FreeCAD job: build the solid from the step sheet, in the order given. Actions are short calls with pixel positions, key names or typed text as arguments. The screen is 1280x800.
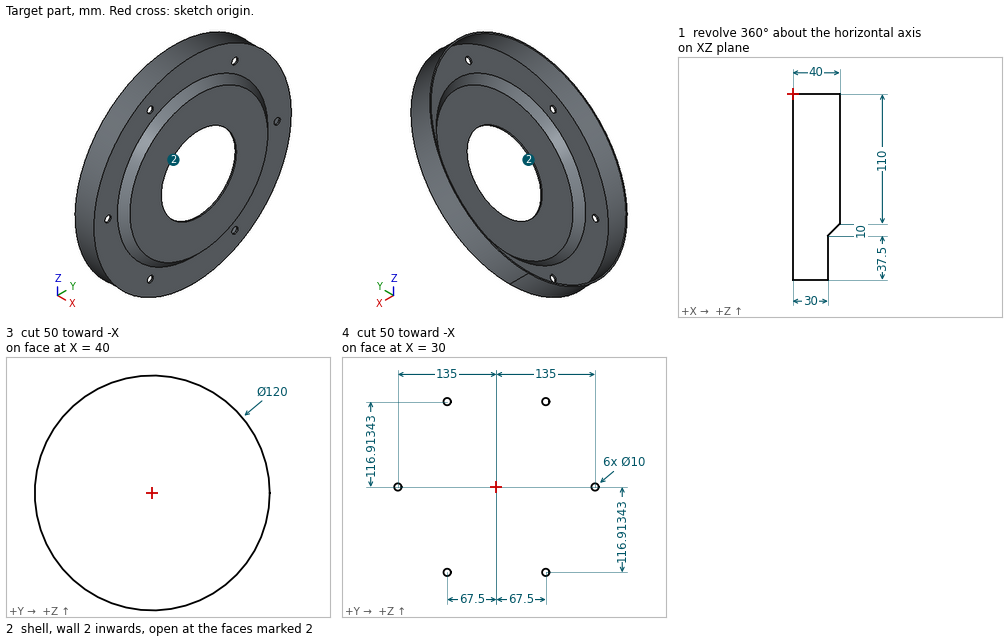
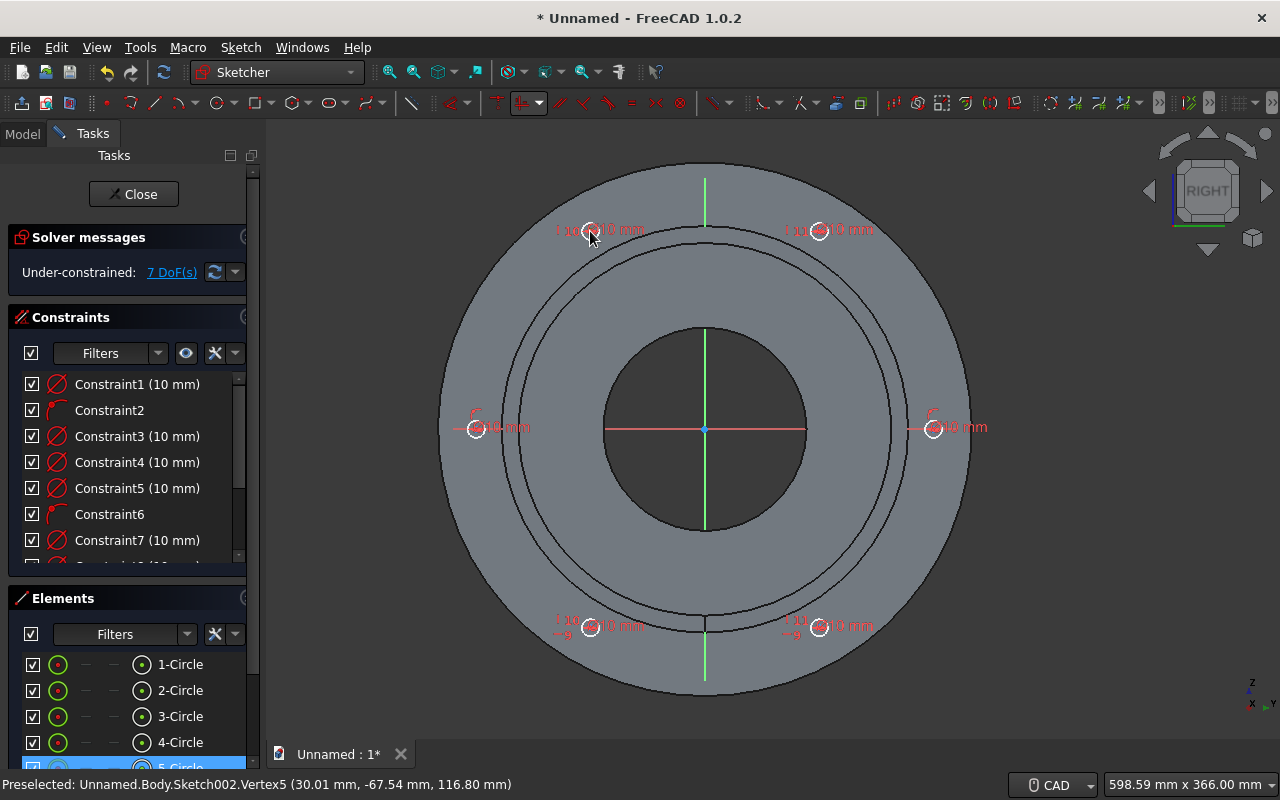
click(819, 231)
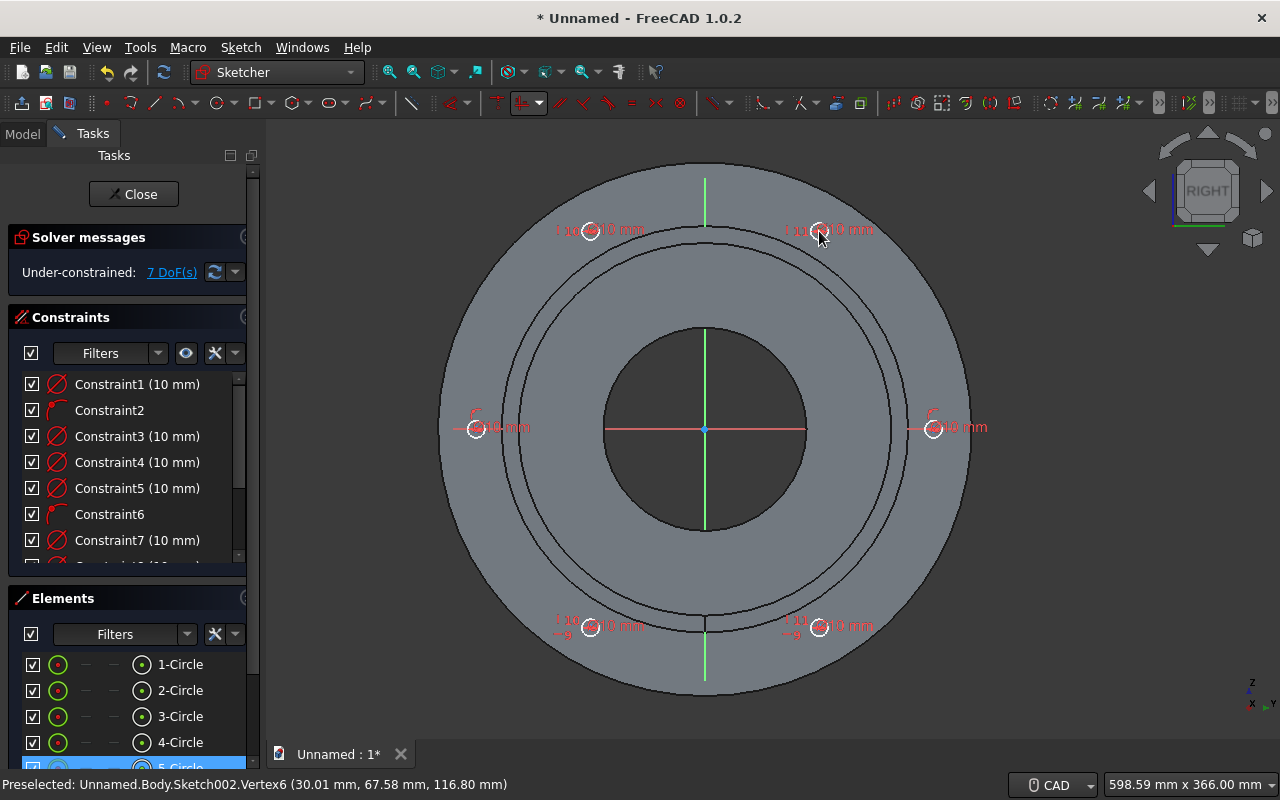
click(542, 104)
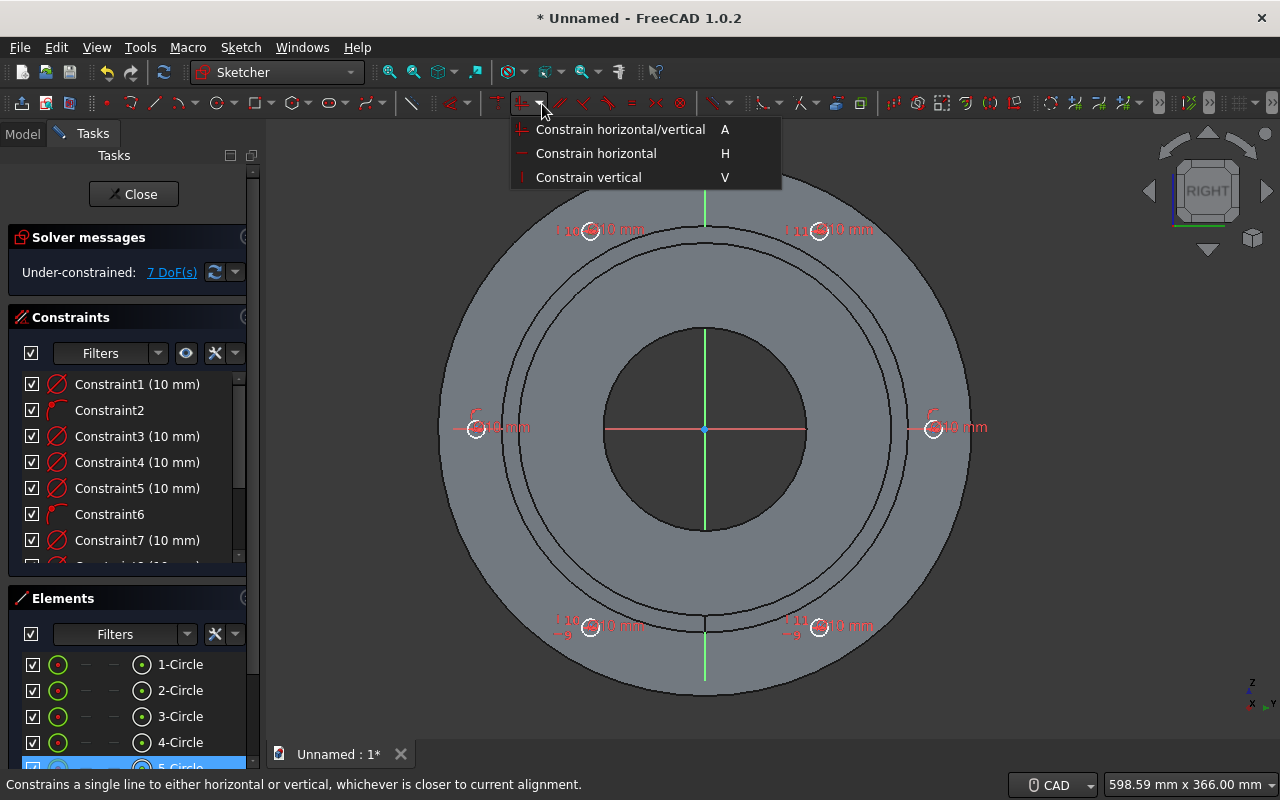
click(646, 153)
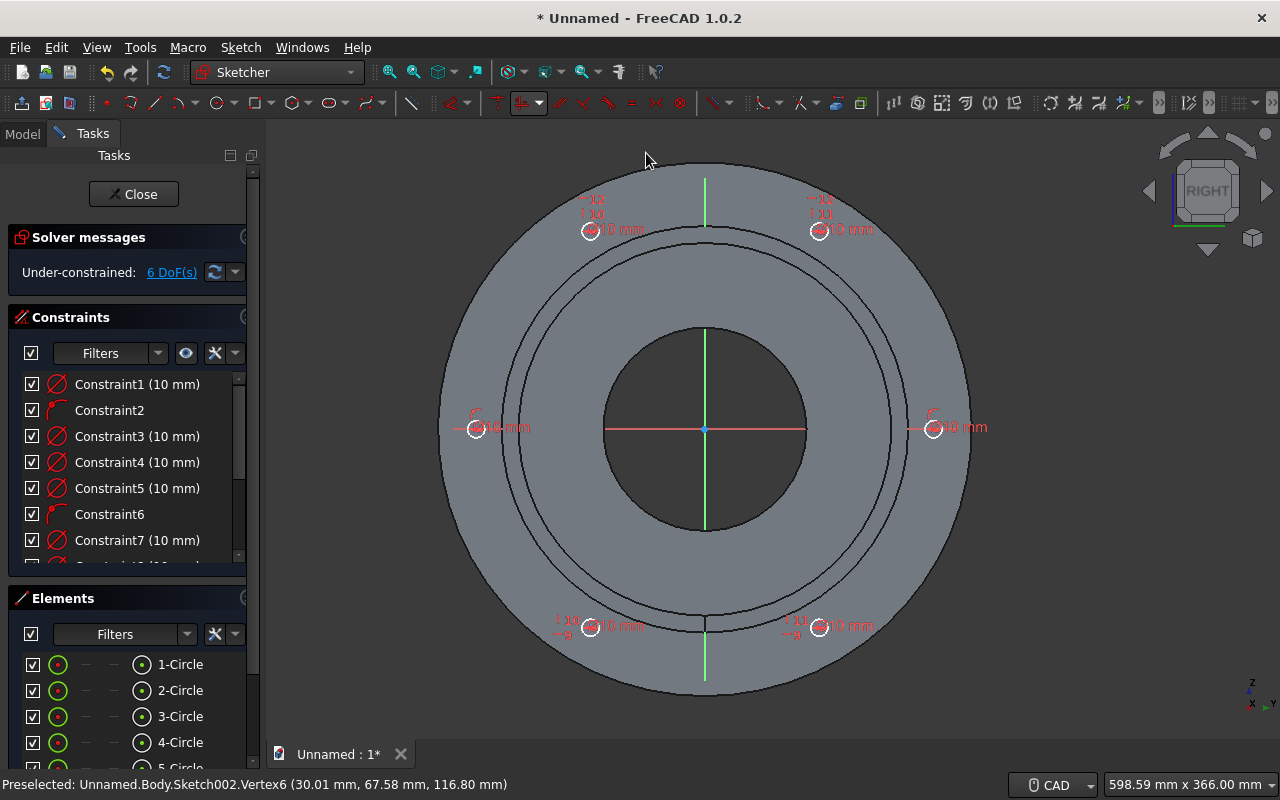
click(450, 104)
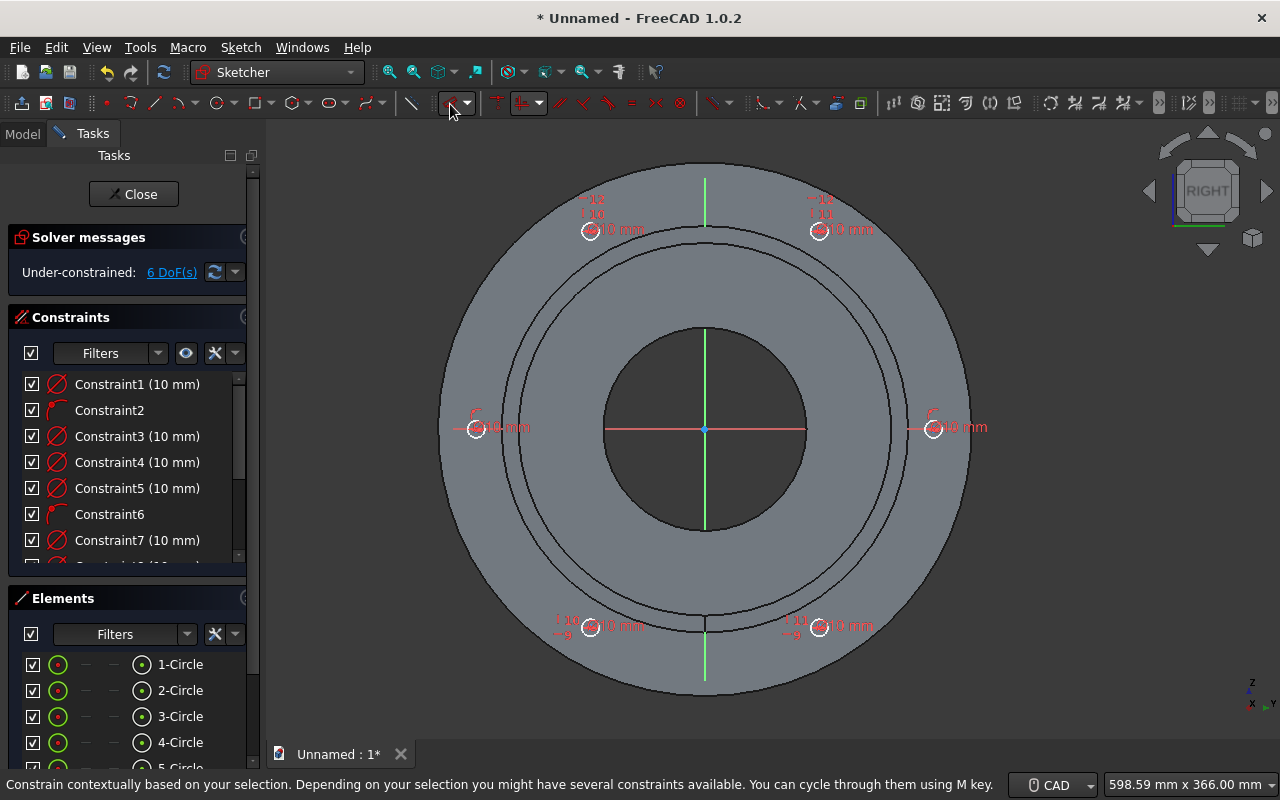
click(933, 429)
click(819, 463)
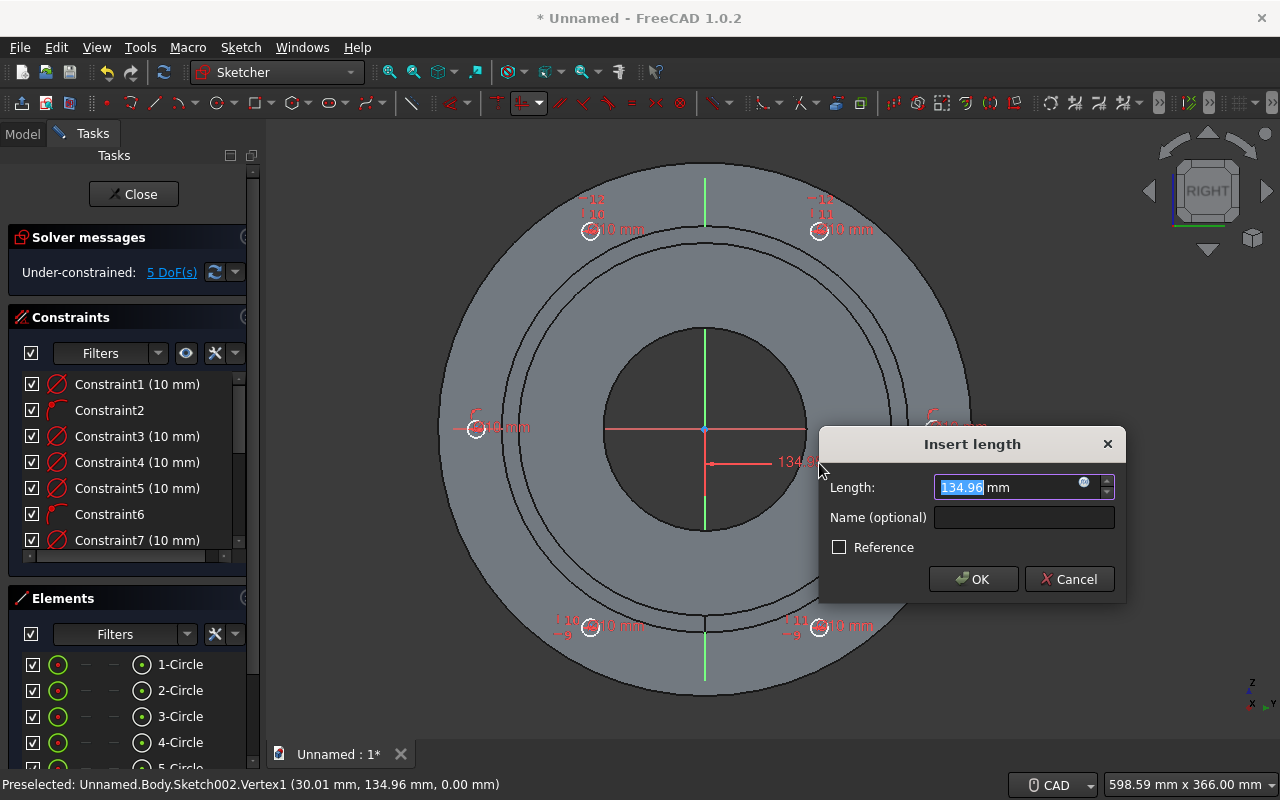
text(135)
key(Return)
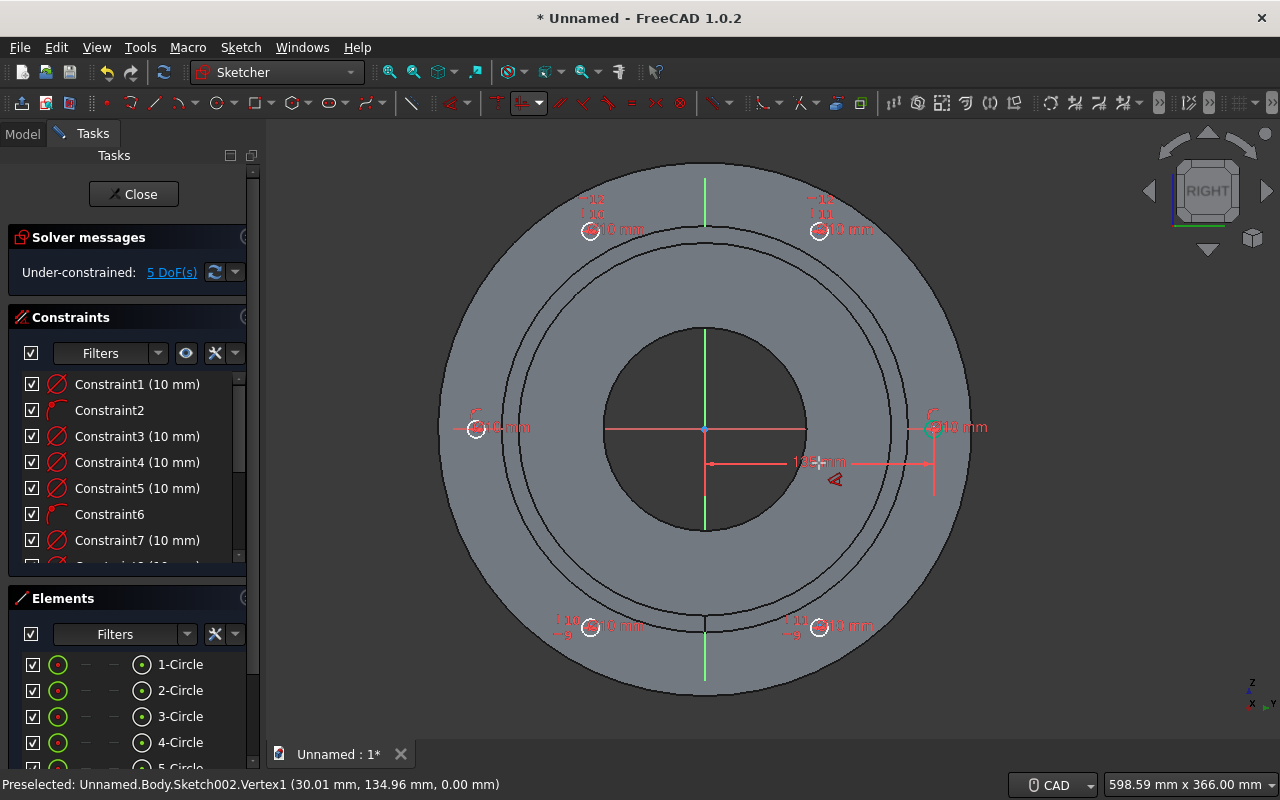
click(476, 429)
click(591, 463)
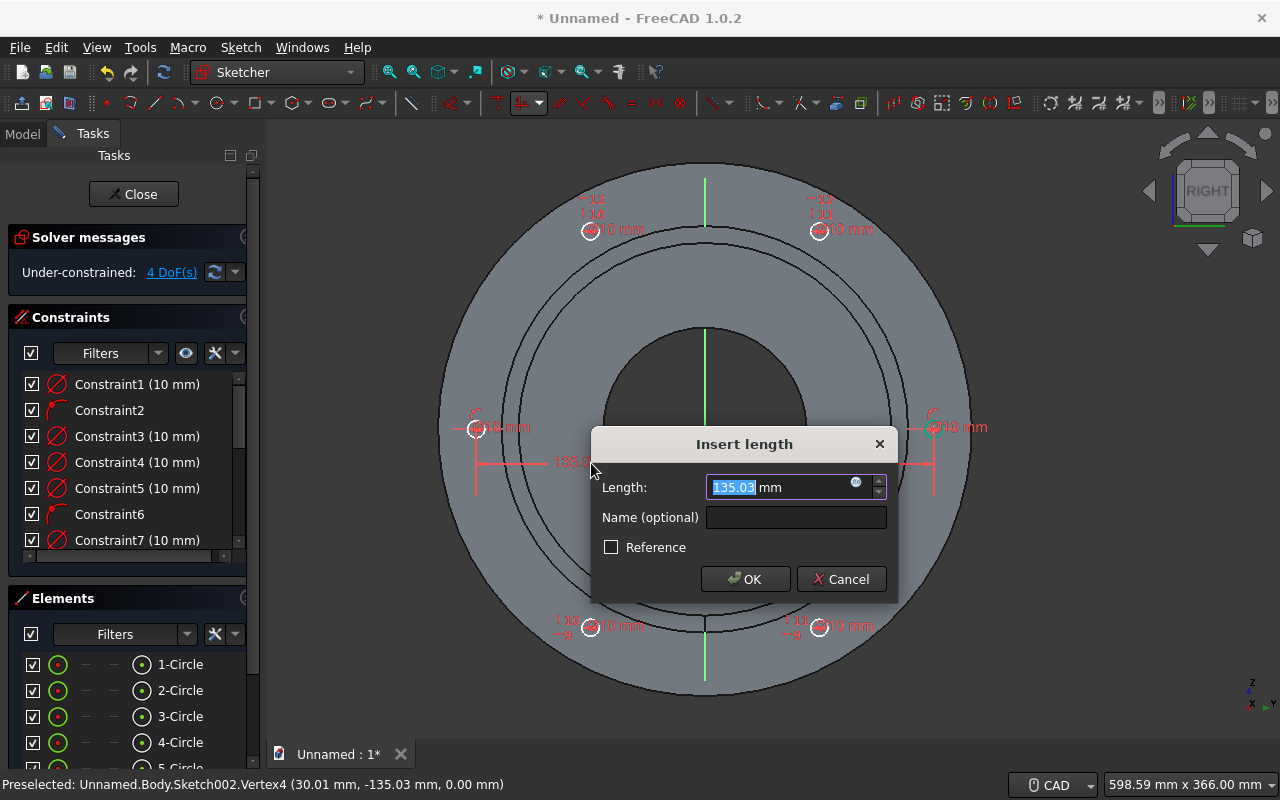
text(135)
key(Return)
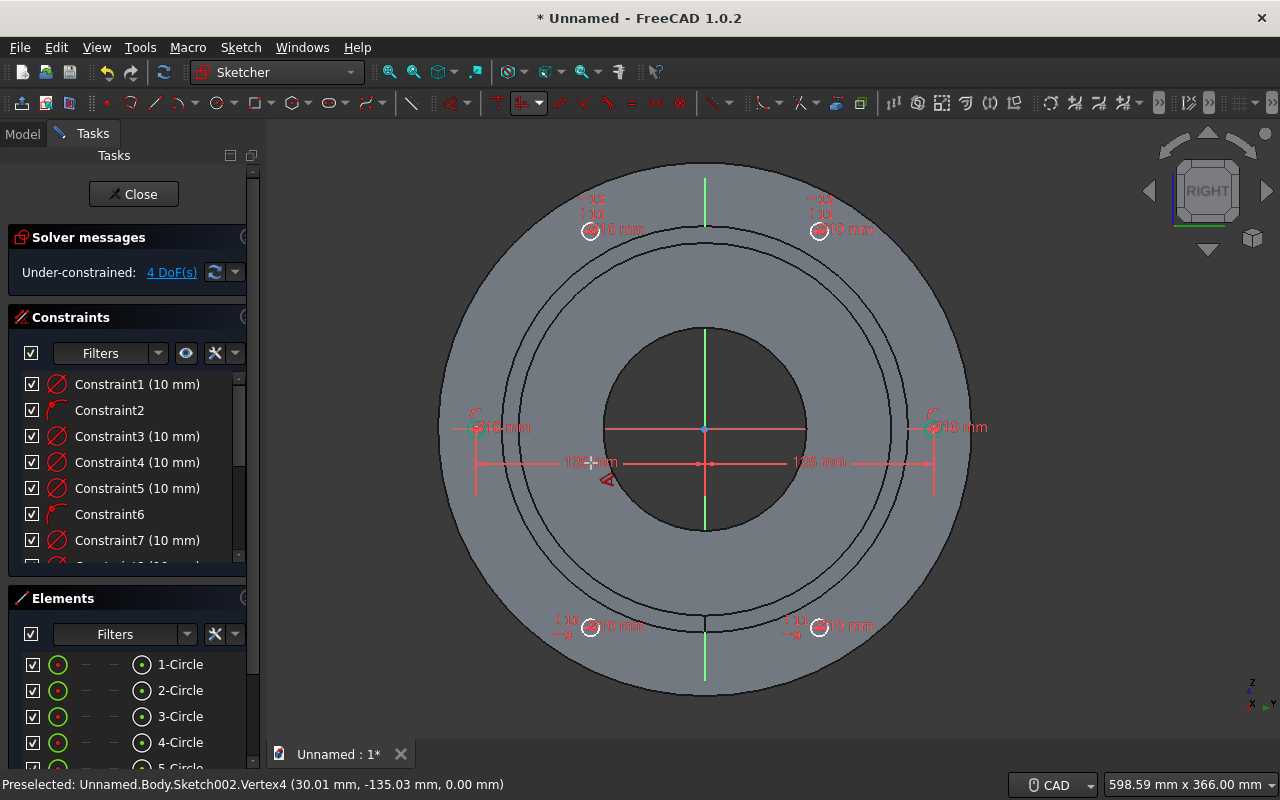
click(819, 628)
click(762, 662)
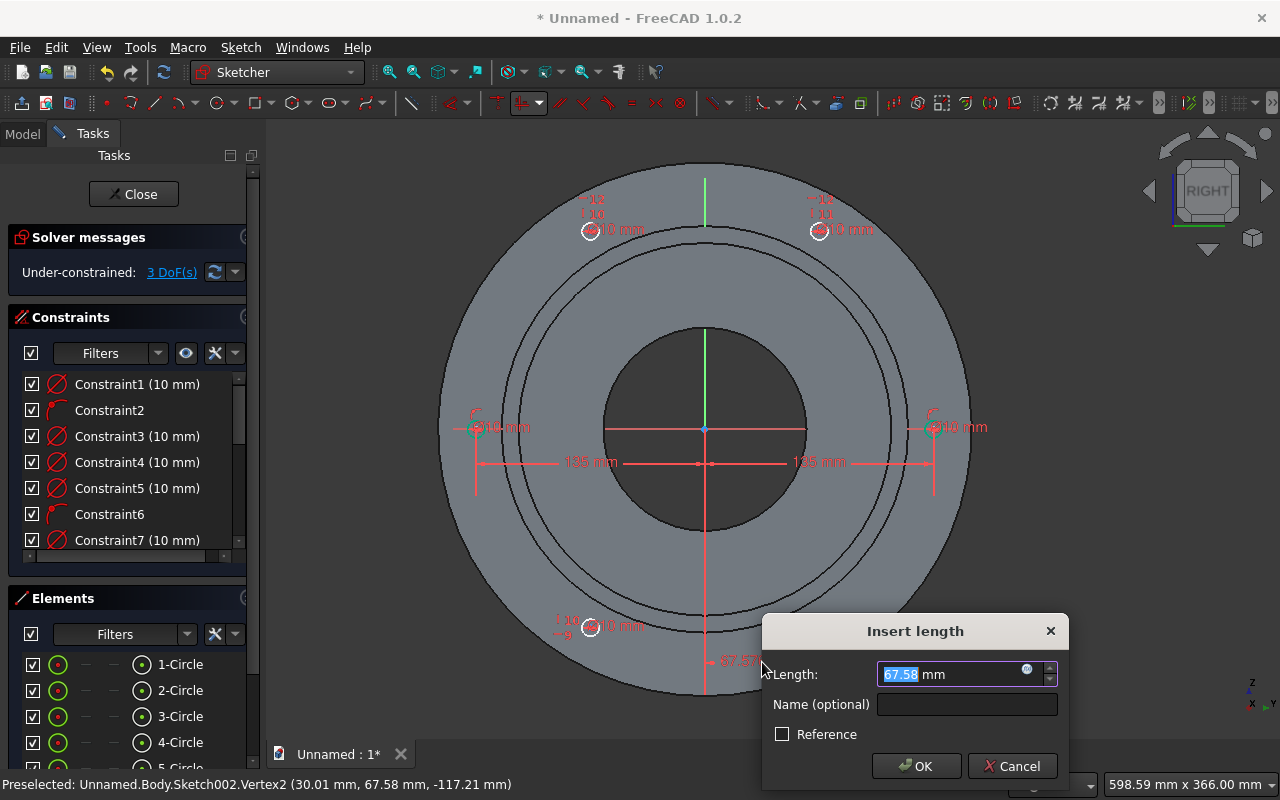
text(67.5)
key(Return)